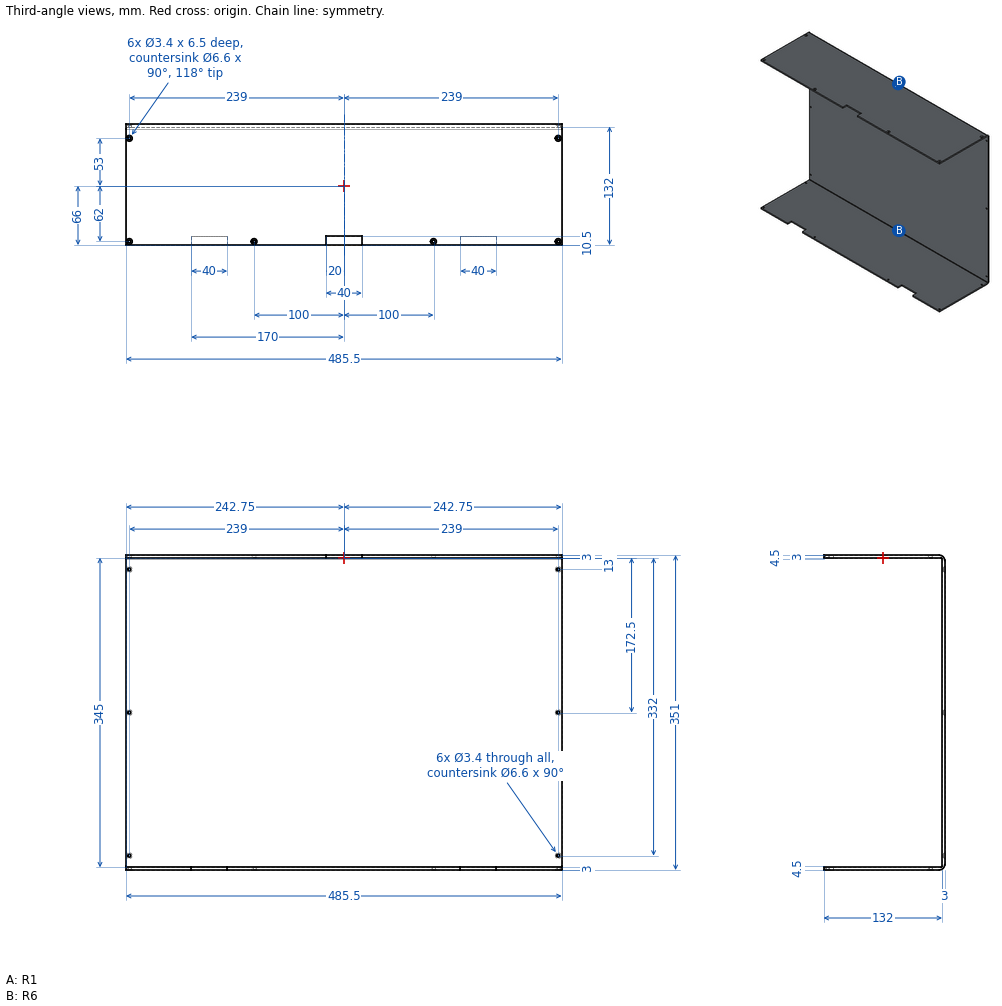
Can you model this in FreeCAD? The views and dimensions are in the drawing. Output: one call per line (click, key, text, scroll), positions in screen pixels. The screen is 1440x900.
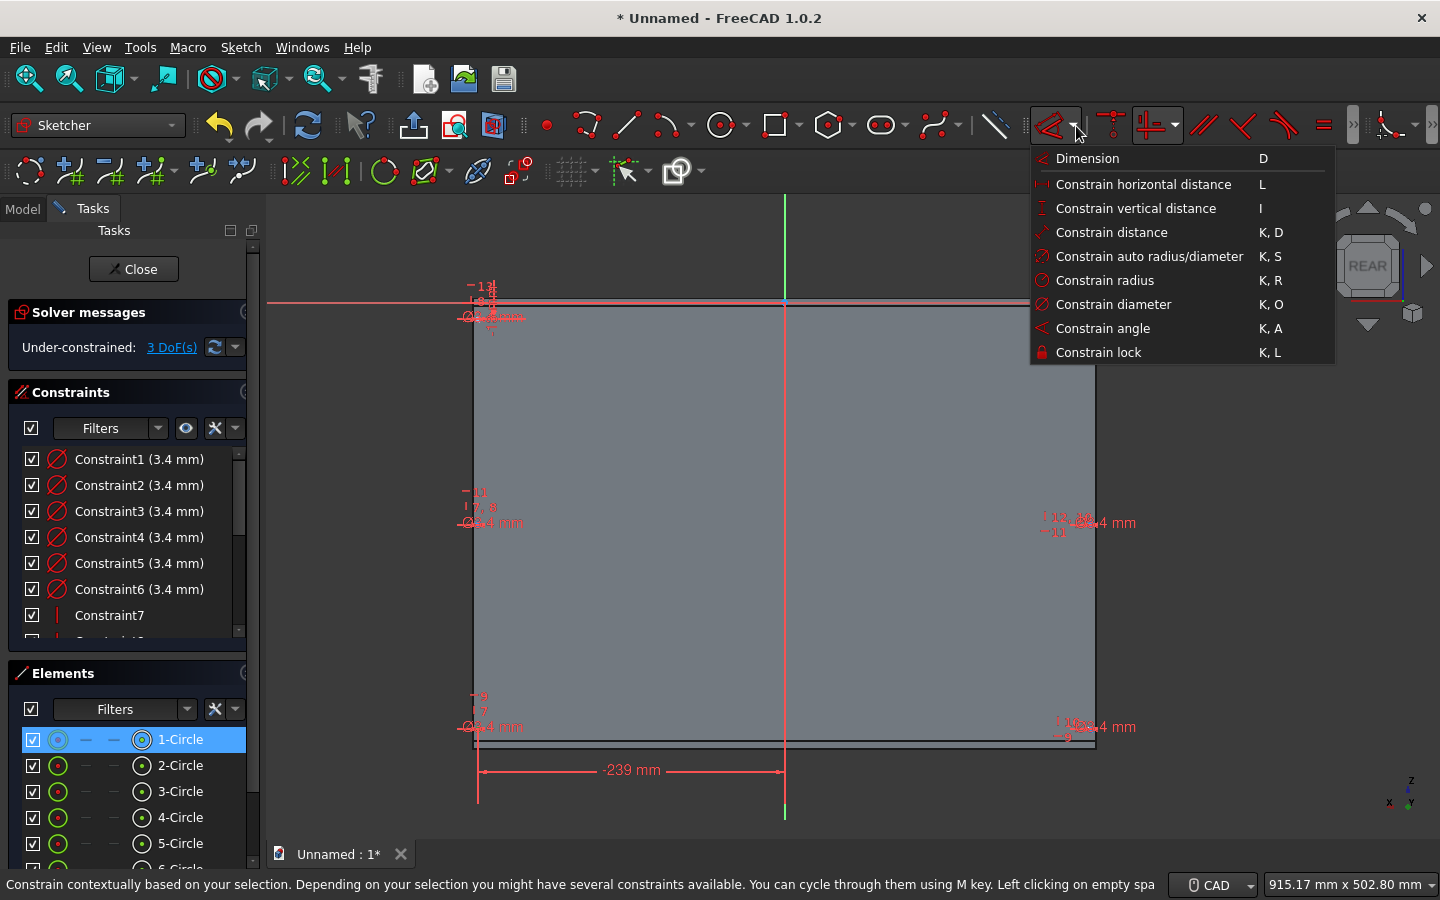
click(1183, 208)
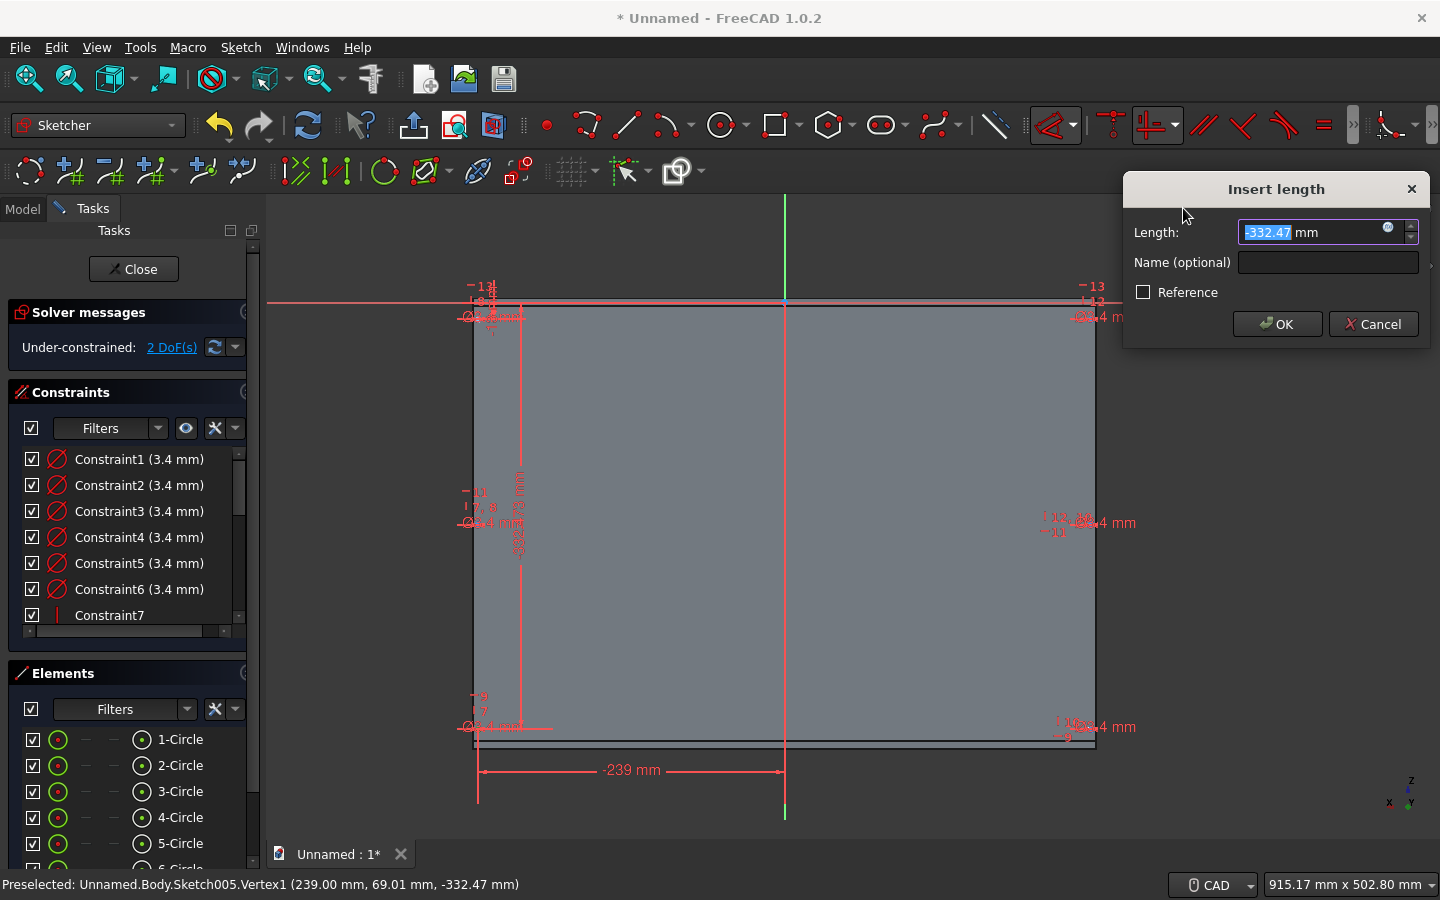
text(-332)
key(Return)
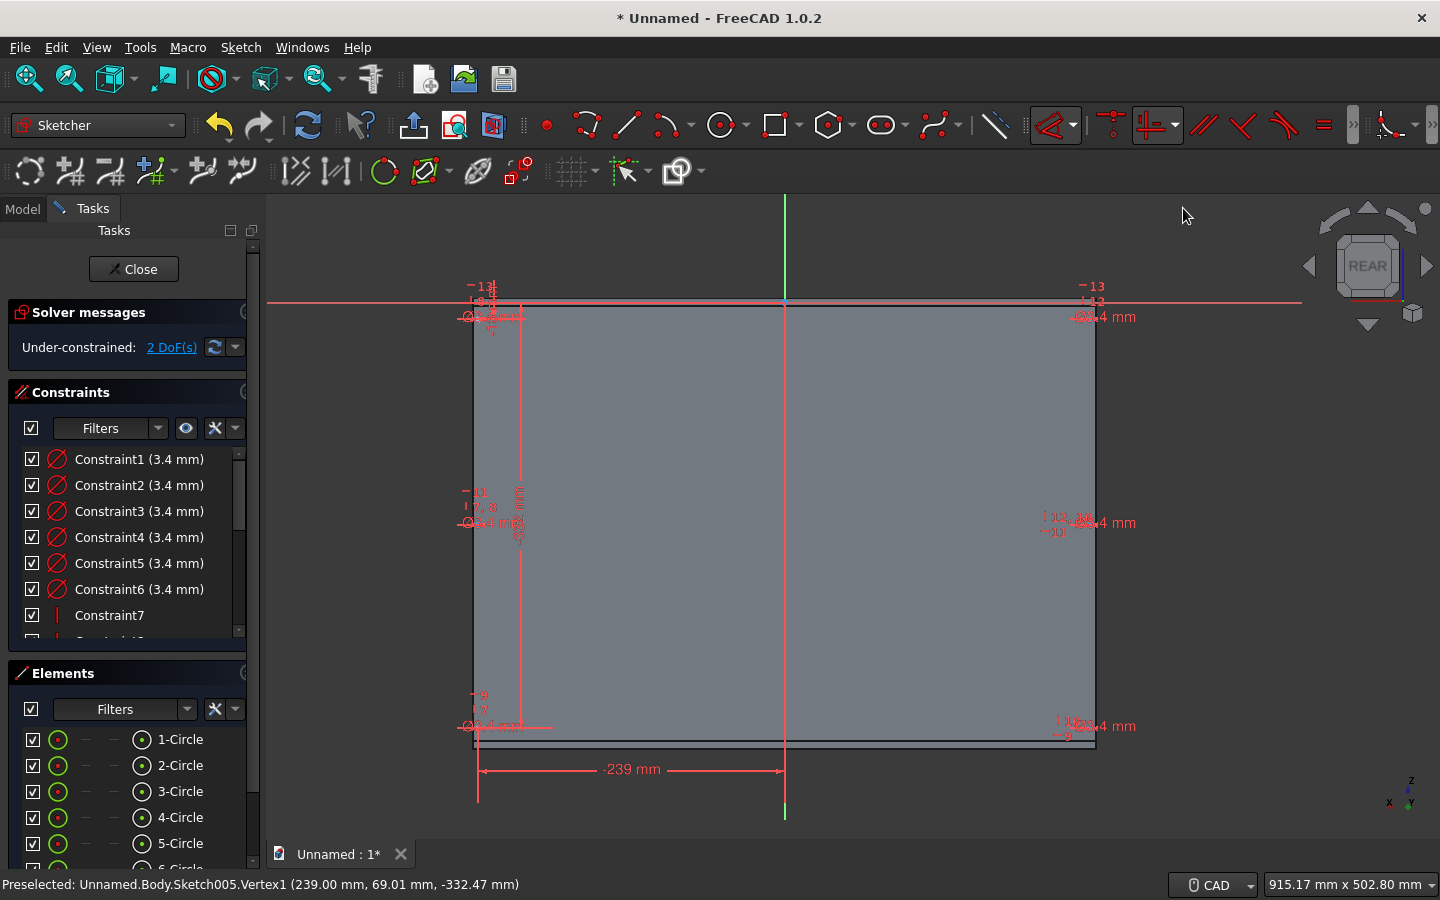
click(1091, 728)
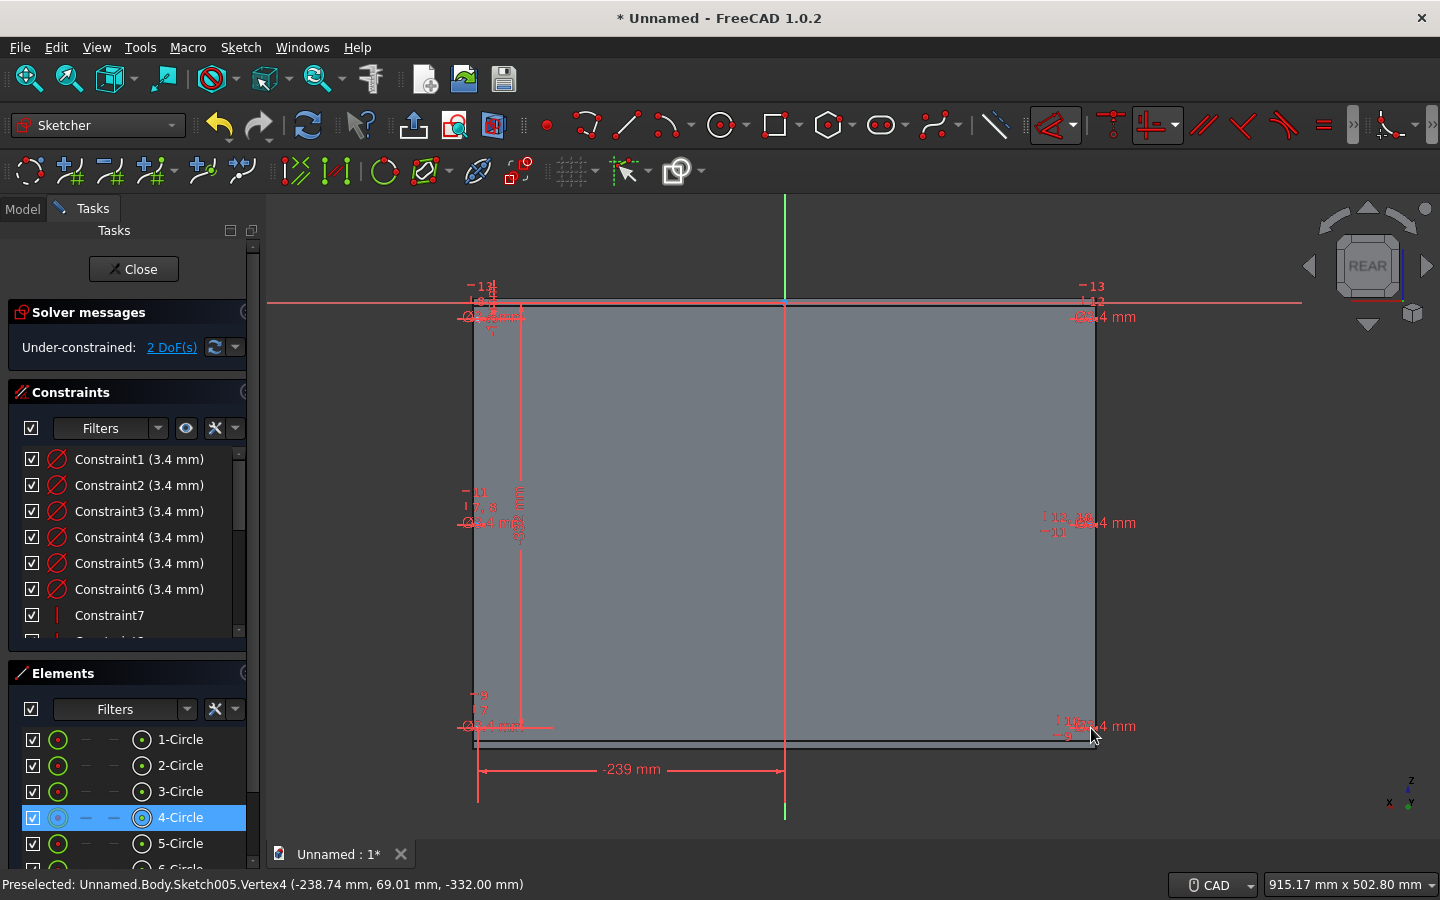
click(1076, 126)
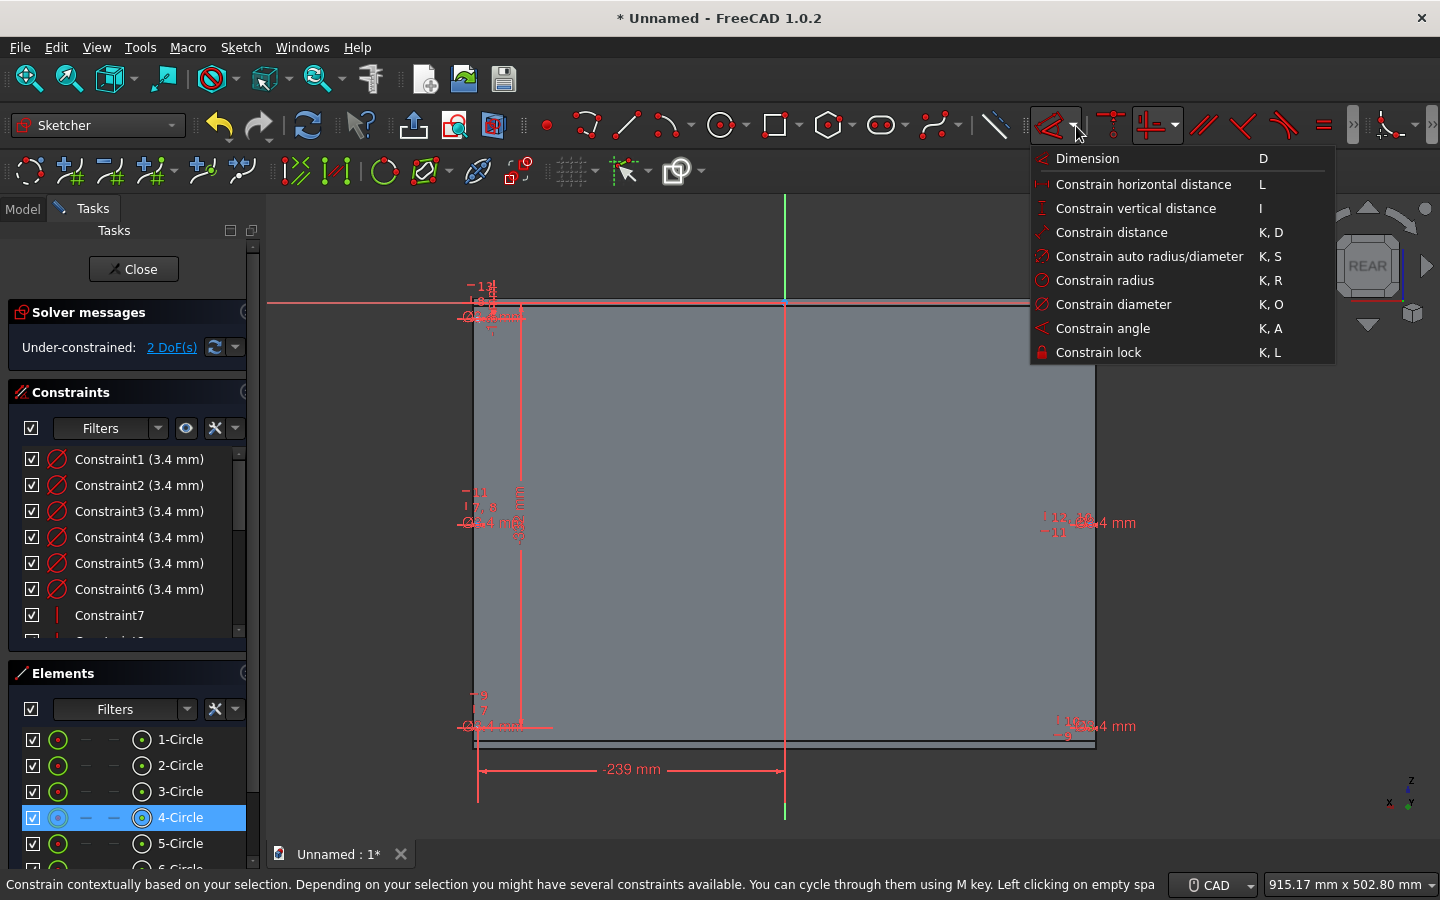
click(1183, 184)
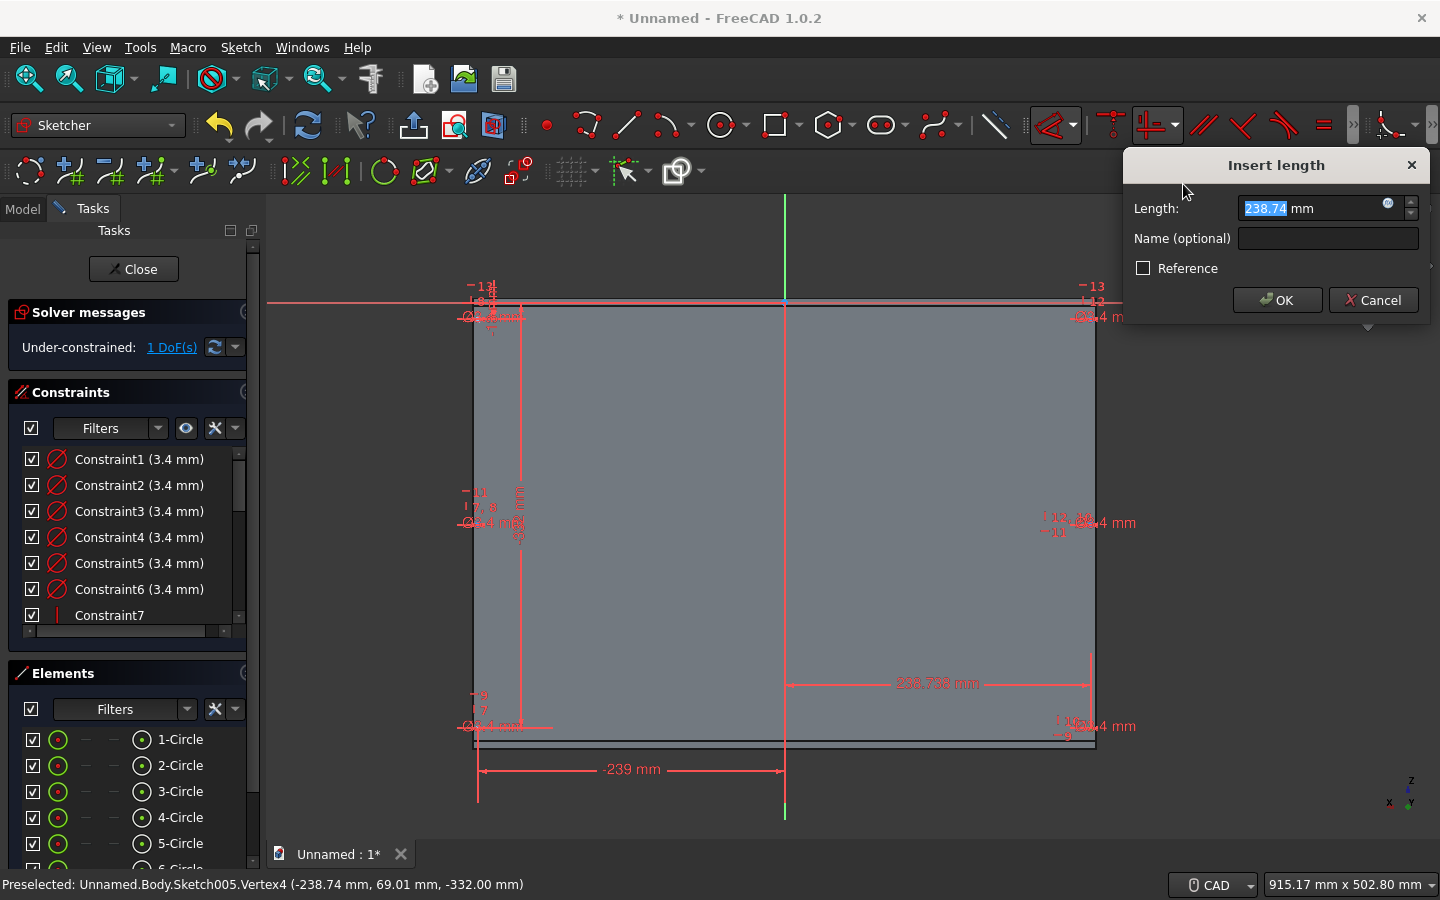
text(239)
key(Return)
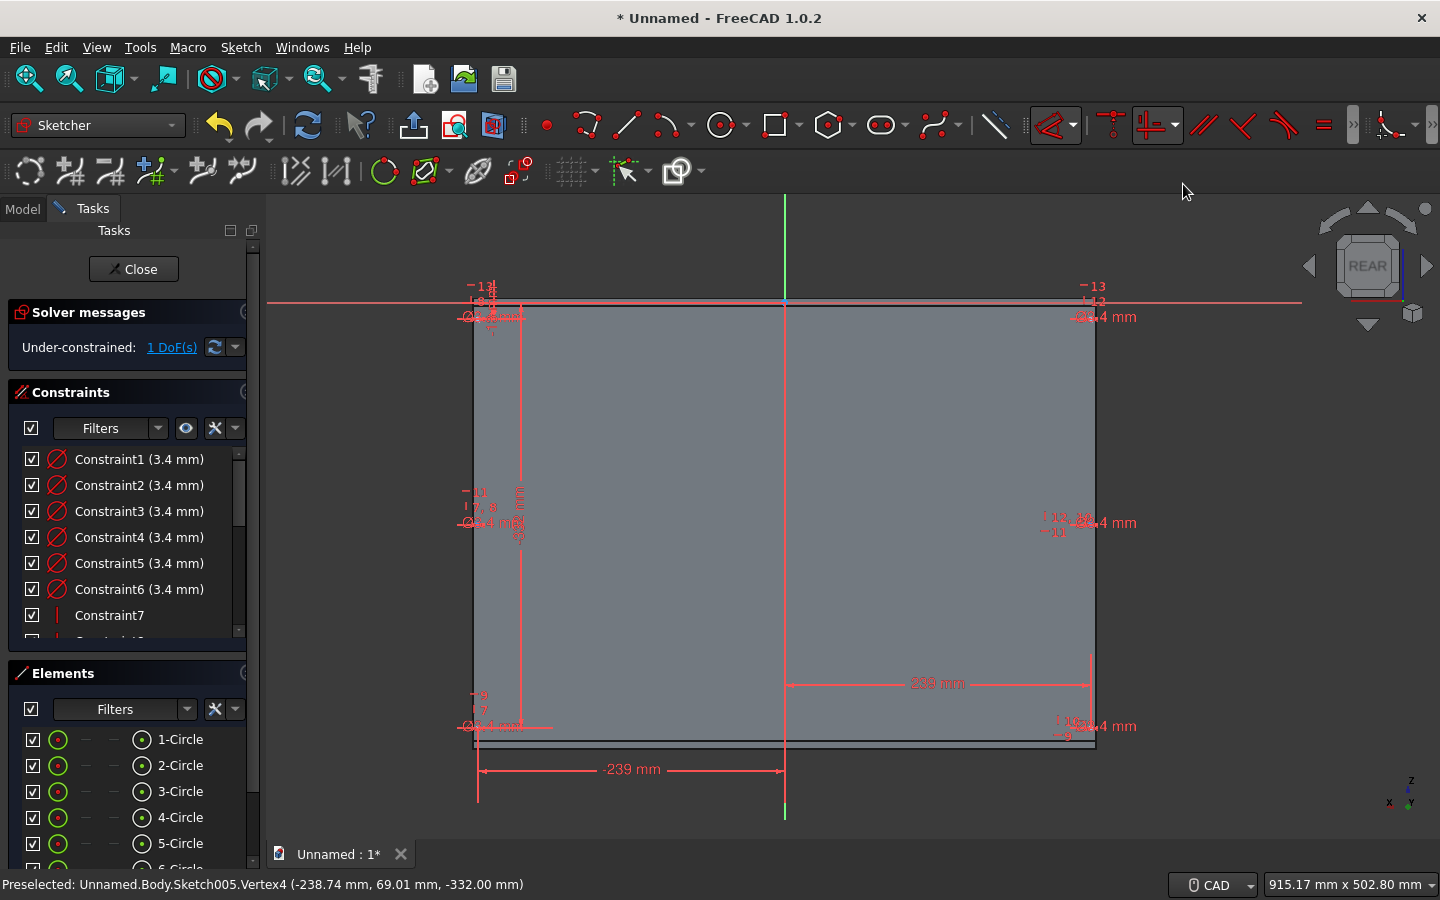
click(478, 525)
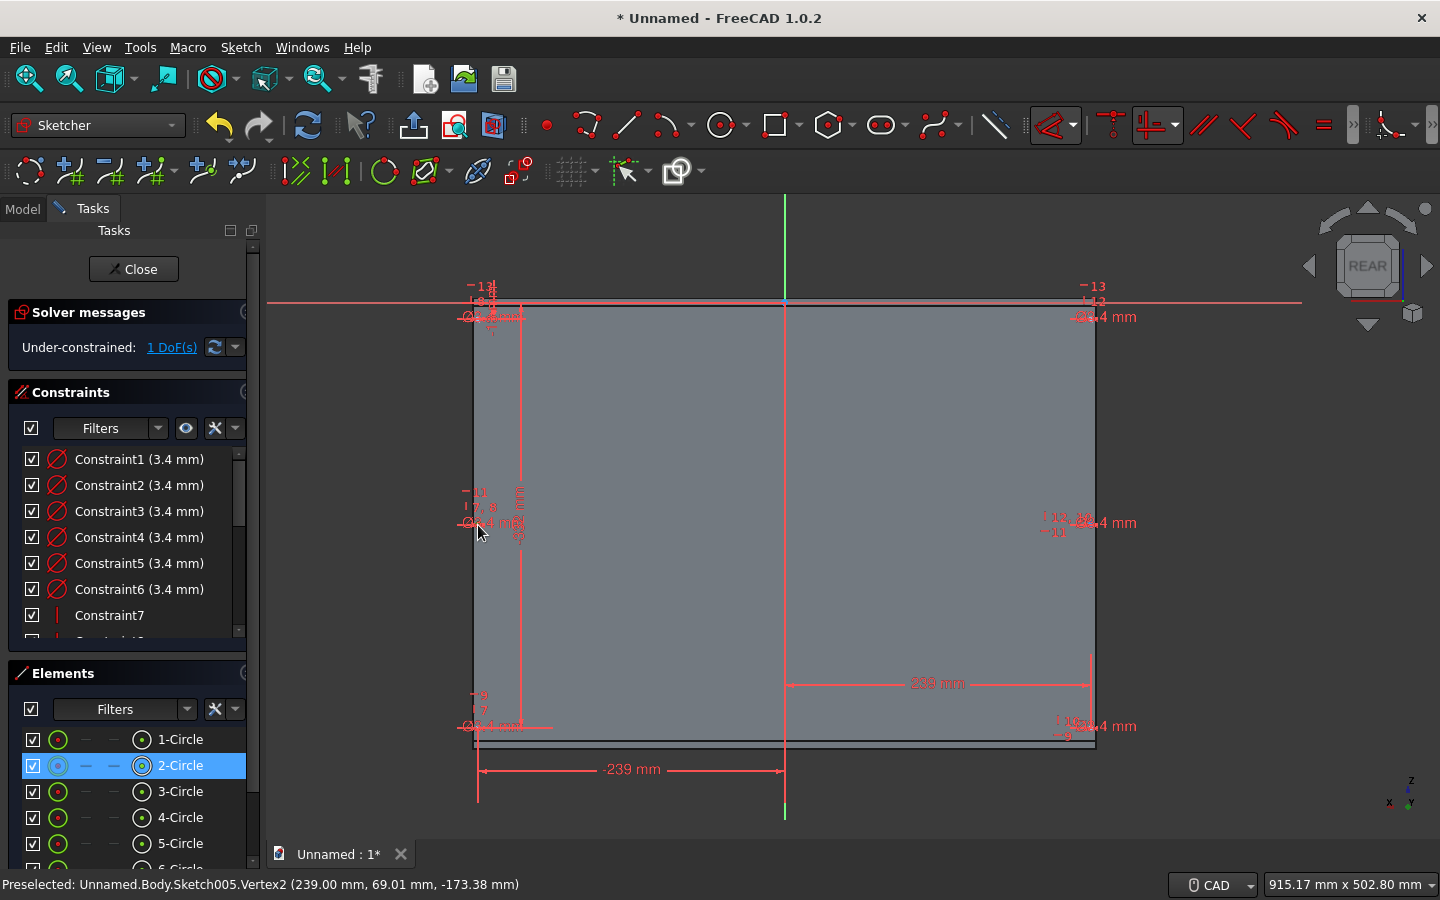
click(1076, 126)